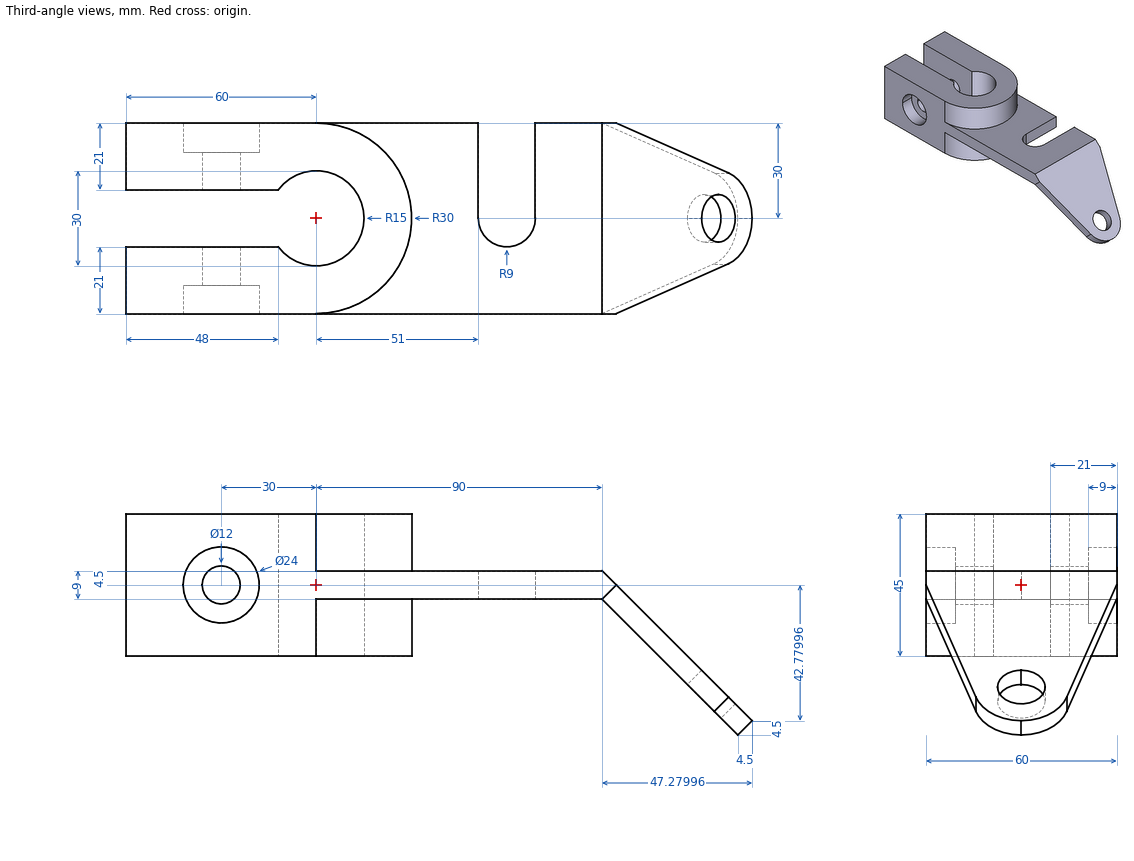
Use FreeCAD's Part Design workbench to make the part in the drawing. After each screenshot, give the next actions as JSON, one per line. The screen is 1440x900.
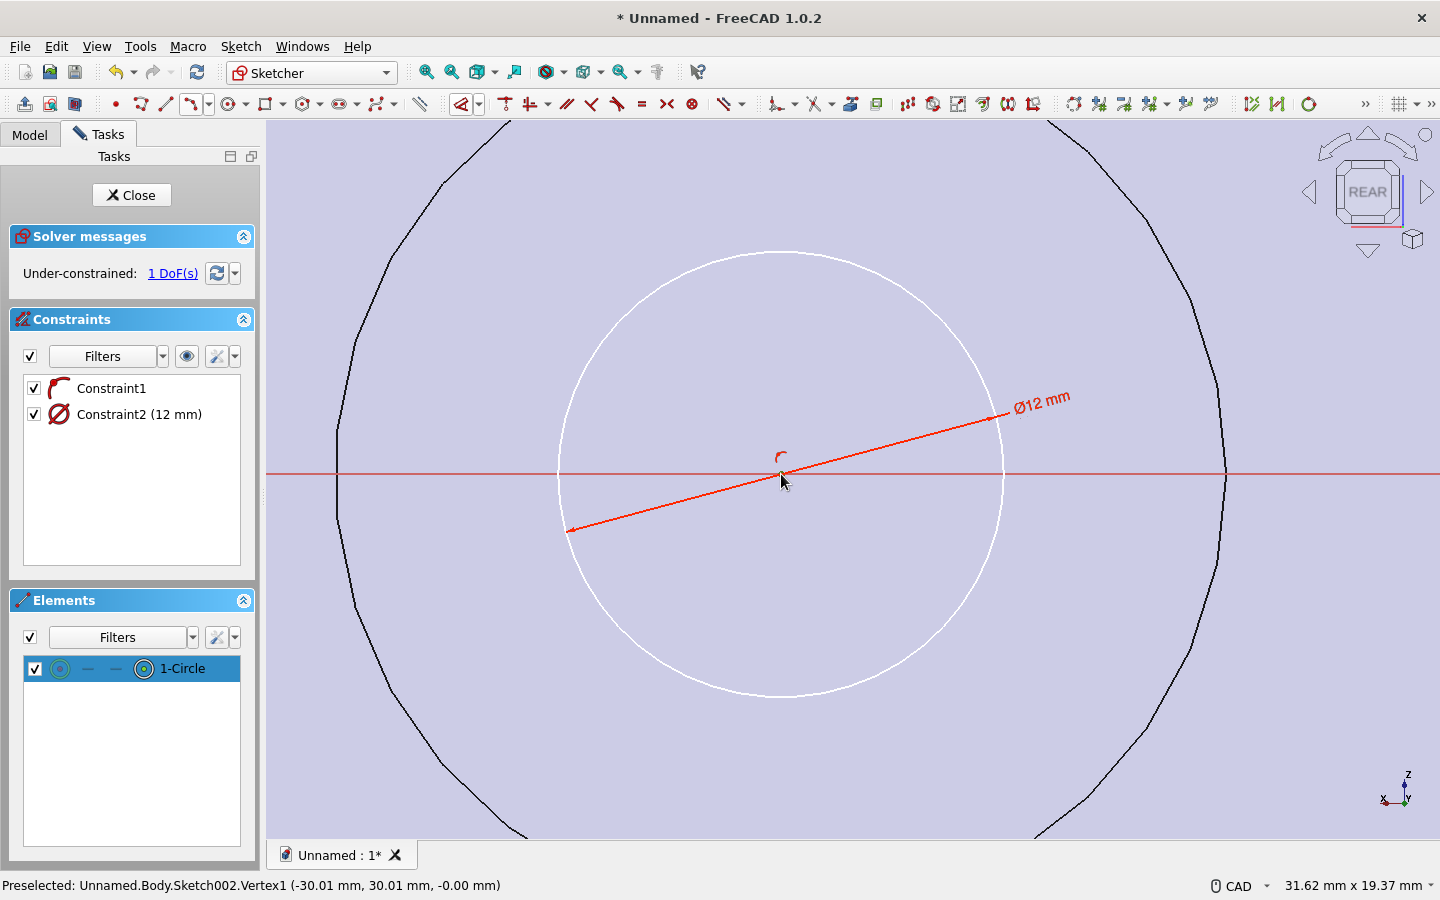
{"action": "key", "text": "l"}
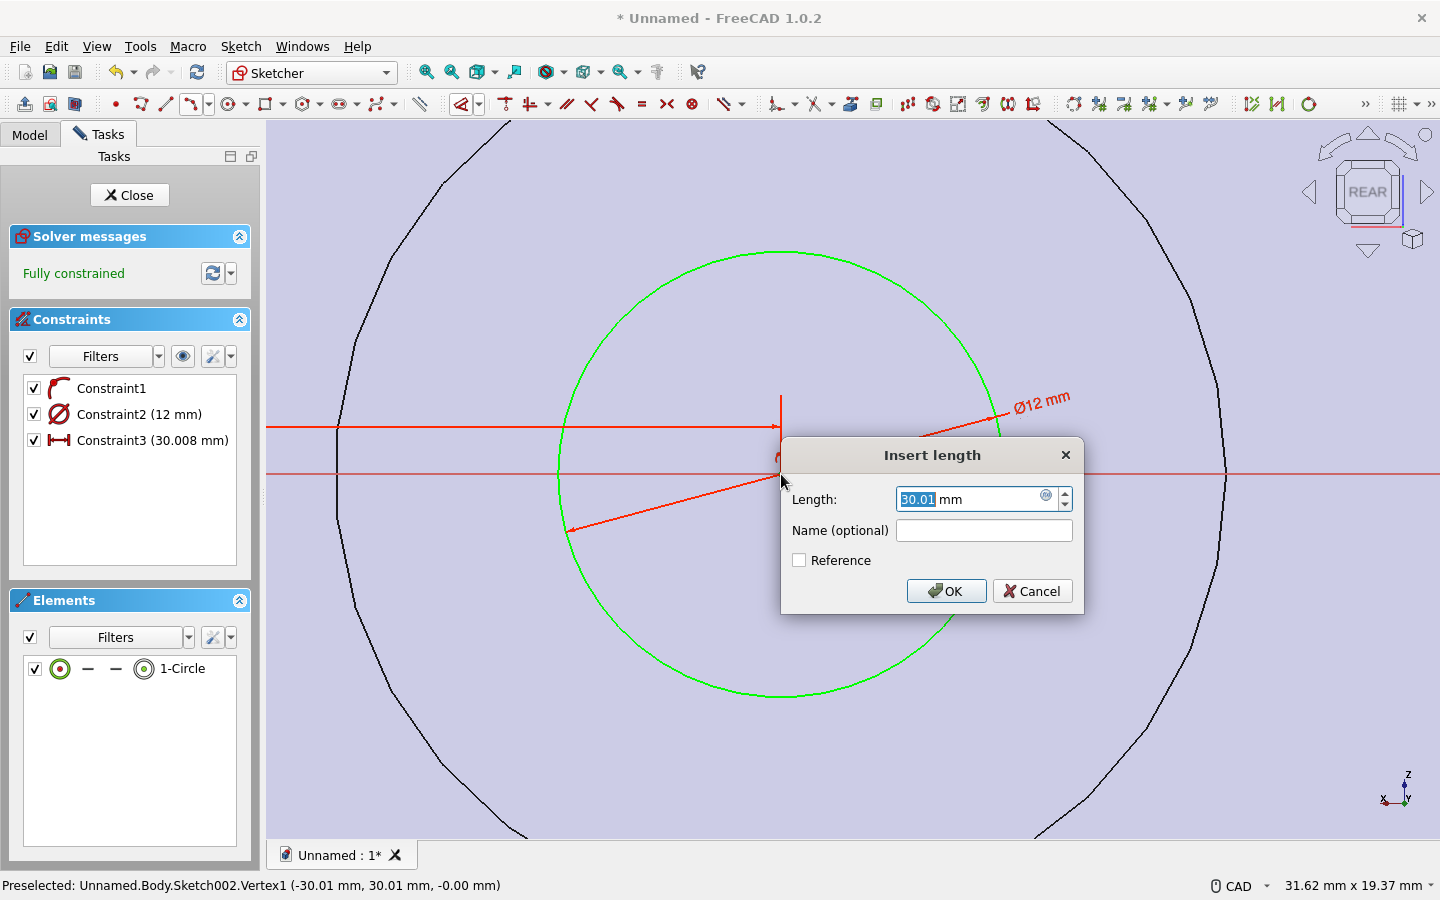
{"action": "type", "text": "30"}
{"action": "key", "text": "Return"}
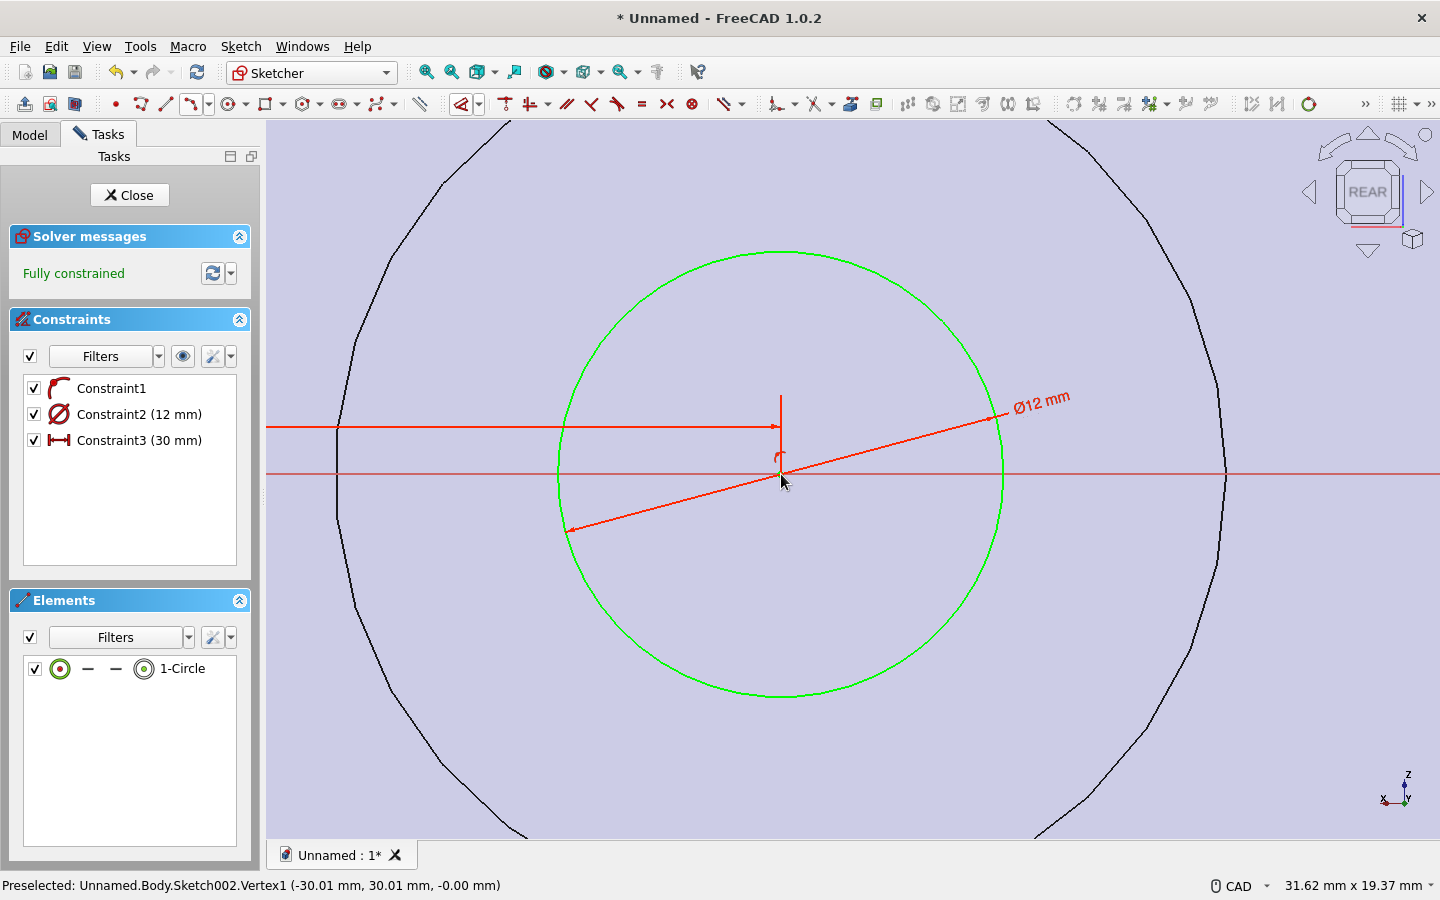
{"action": "left_click", "coordinate": [130, 195]}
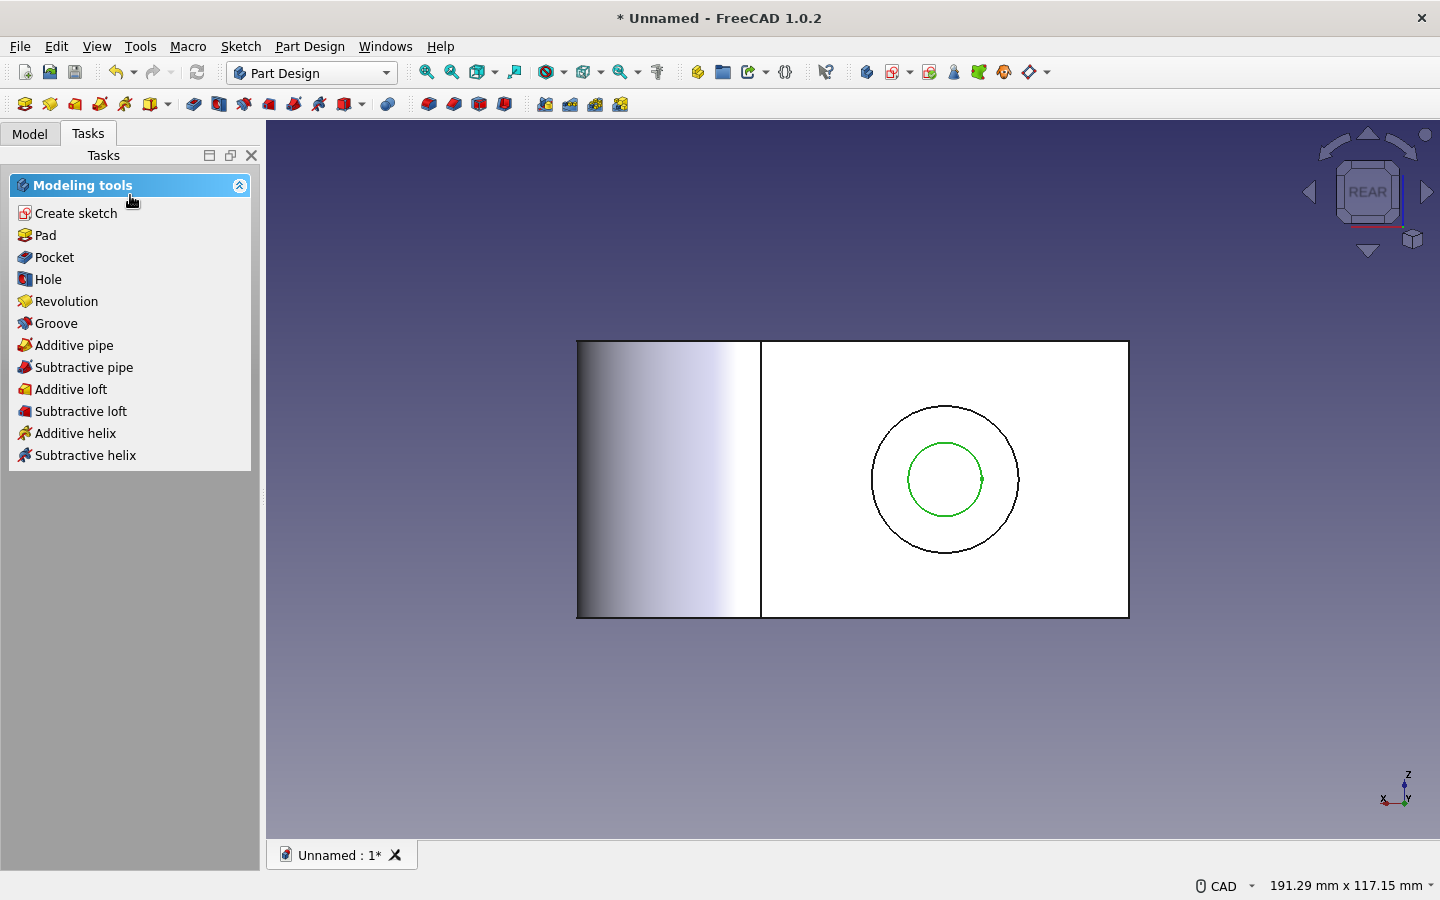
{"action": "left_click", "coordinate": [194, 104]}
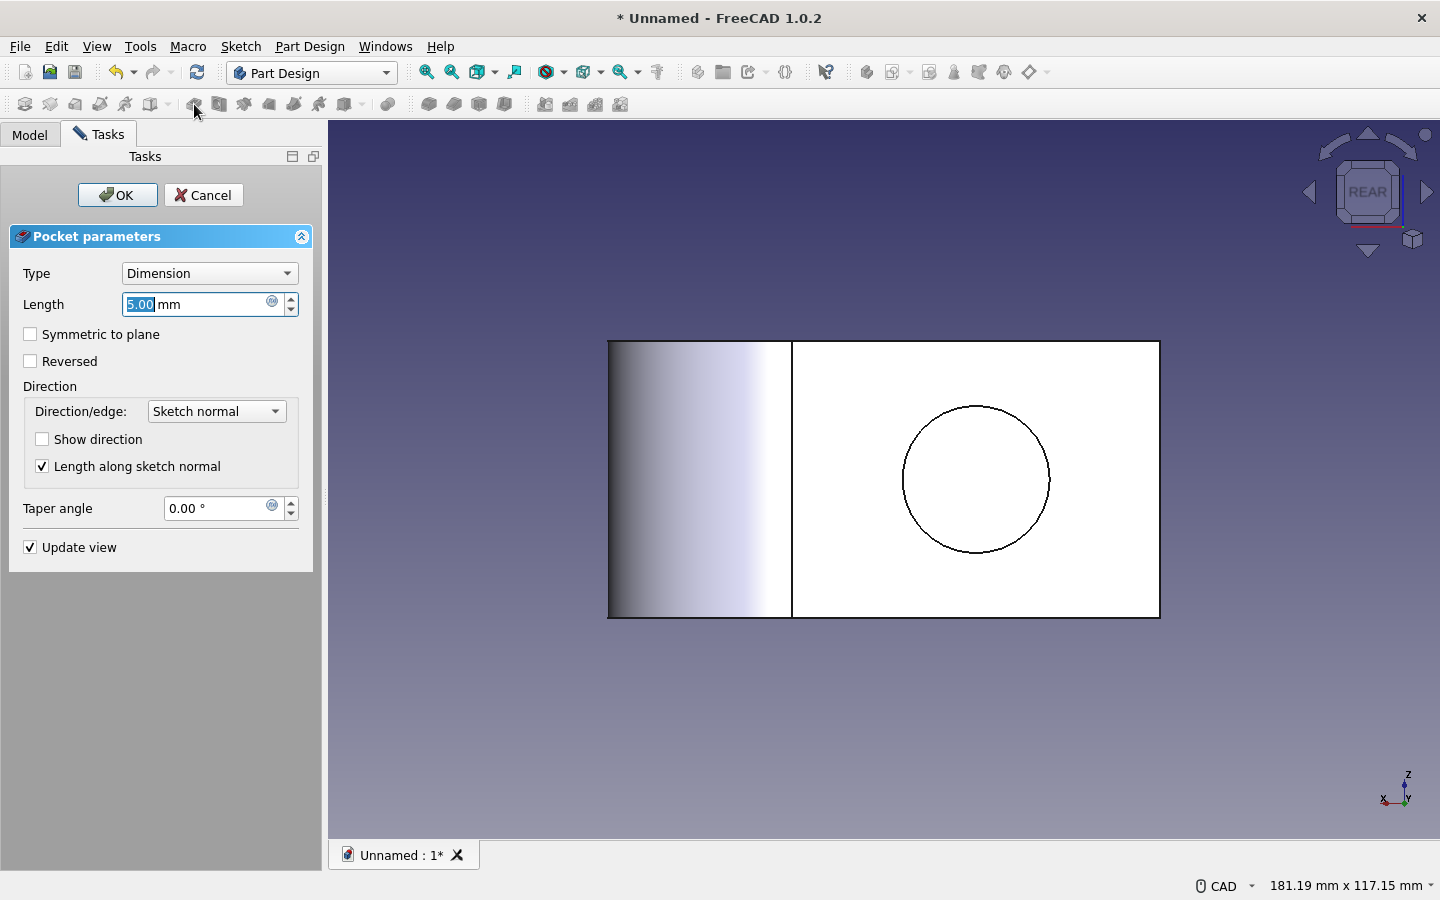
{"action": "type", "text": "21"}
{"action": "key", "text": "Tab"}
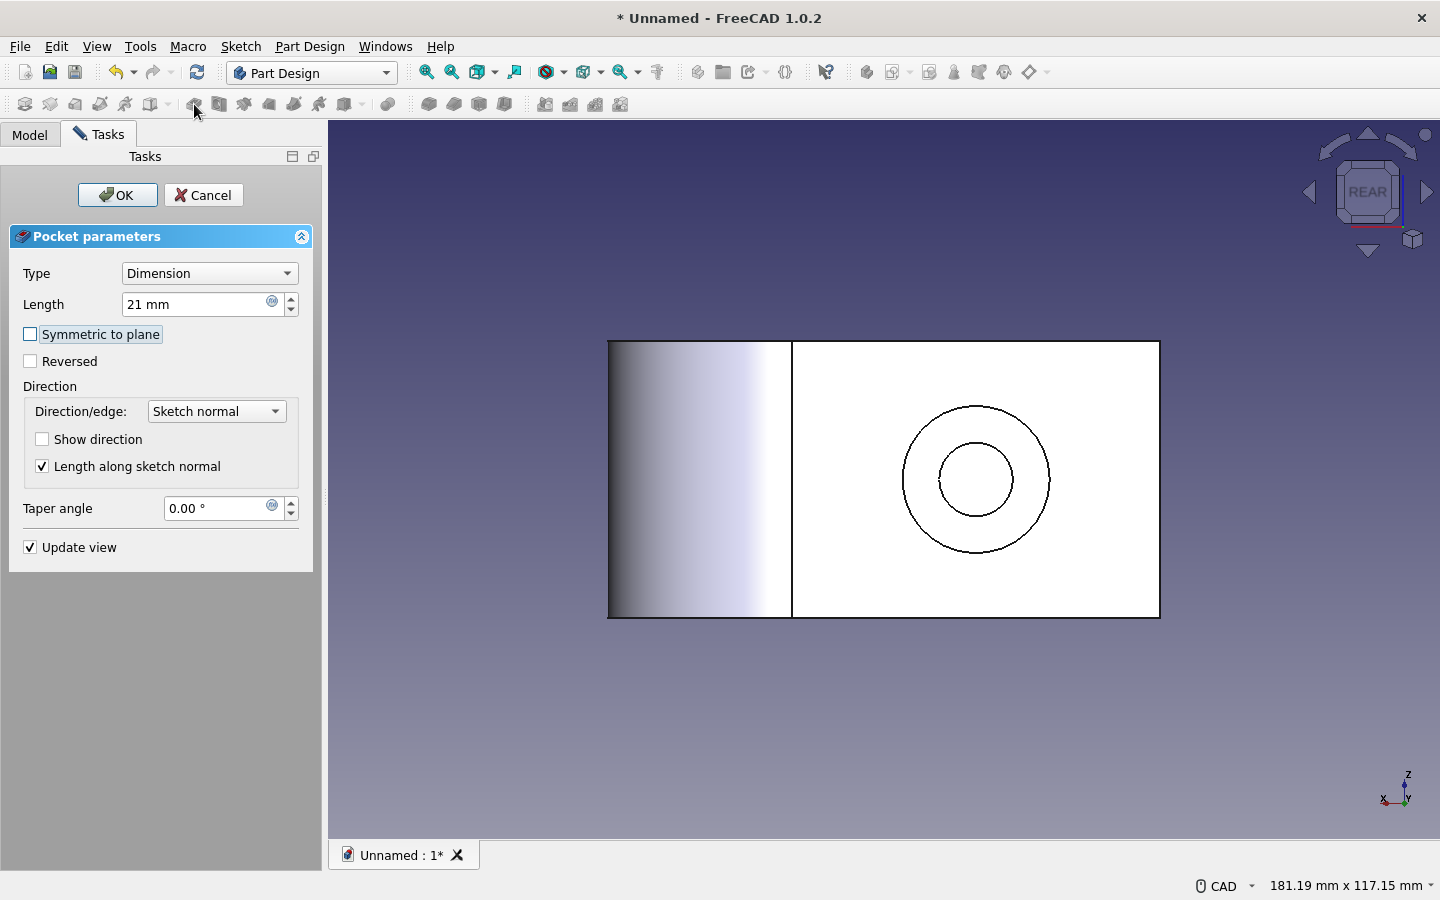
{"action": "left_click", "coordinate": [118, 195]}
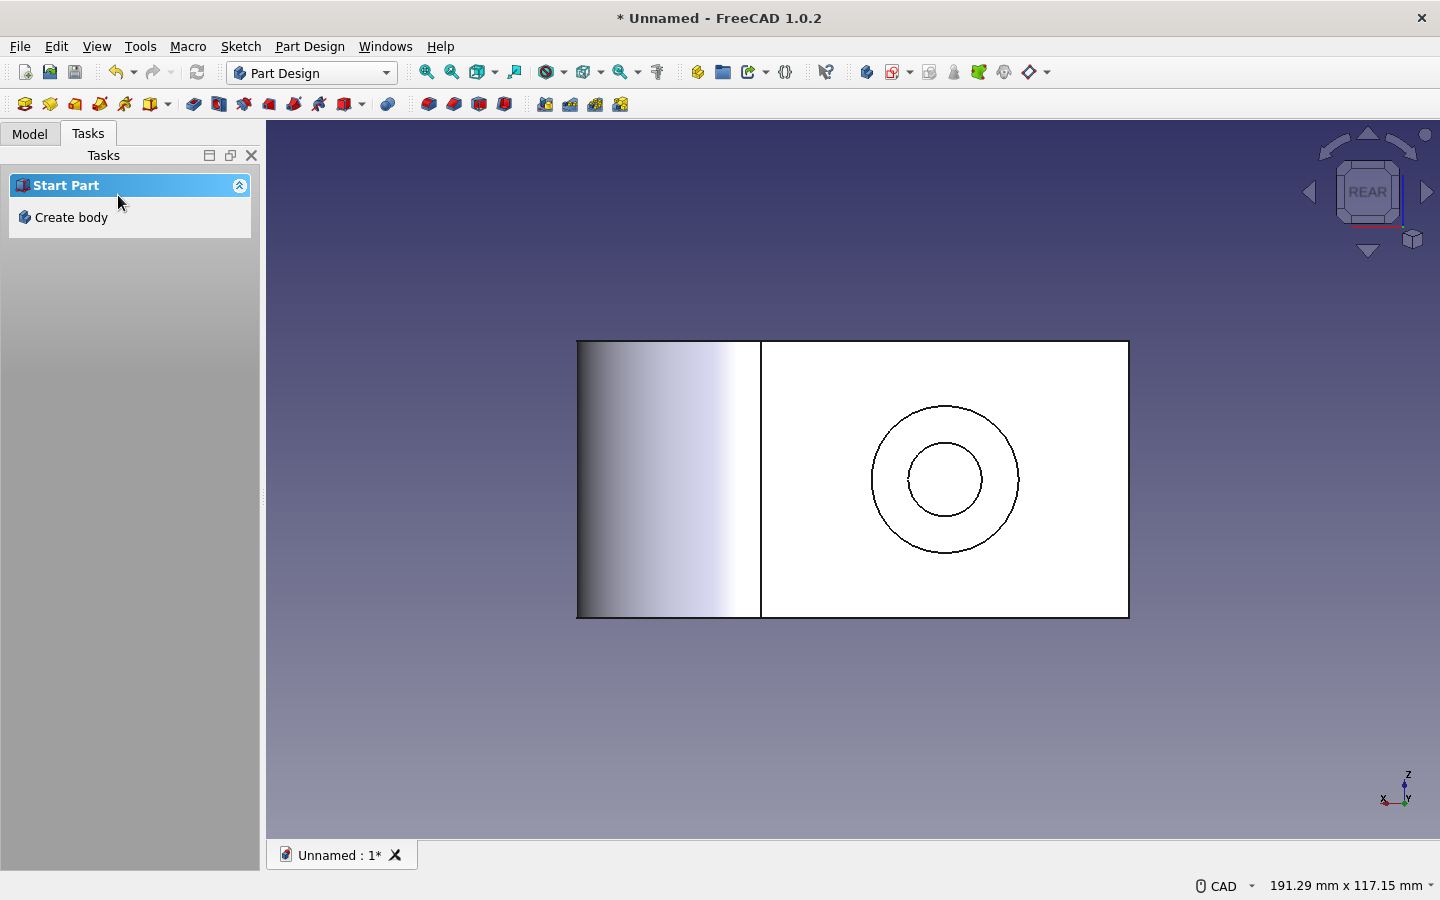
{"action": "left_click", "coordinate": [30, 134]}